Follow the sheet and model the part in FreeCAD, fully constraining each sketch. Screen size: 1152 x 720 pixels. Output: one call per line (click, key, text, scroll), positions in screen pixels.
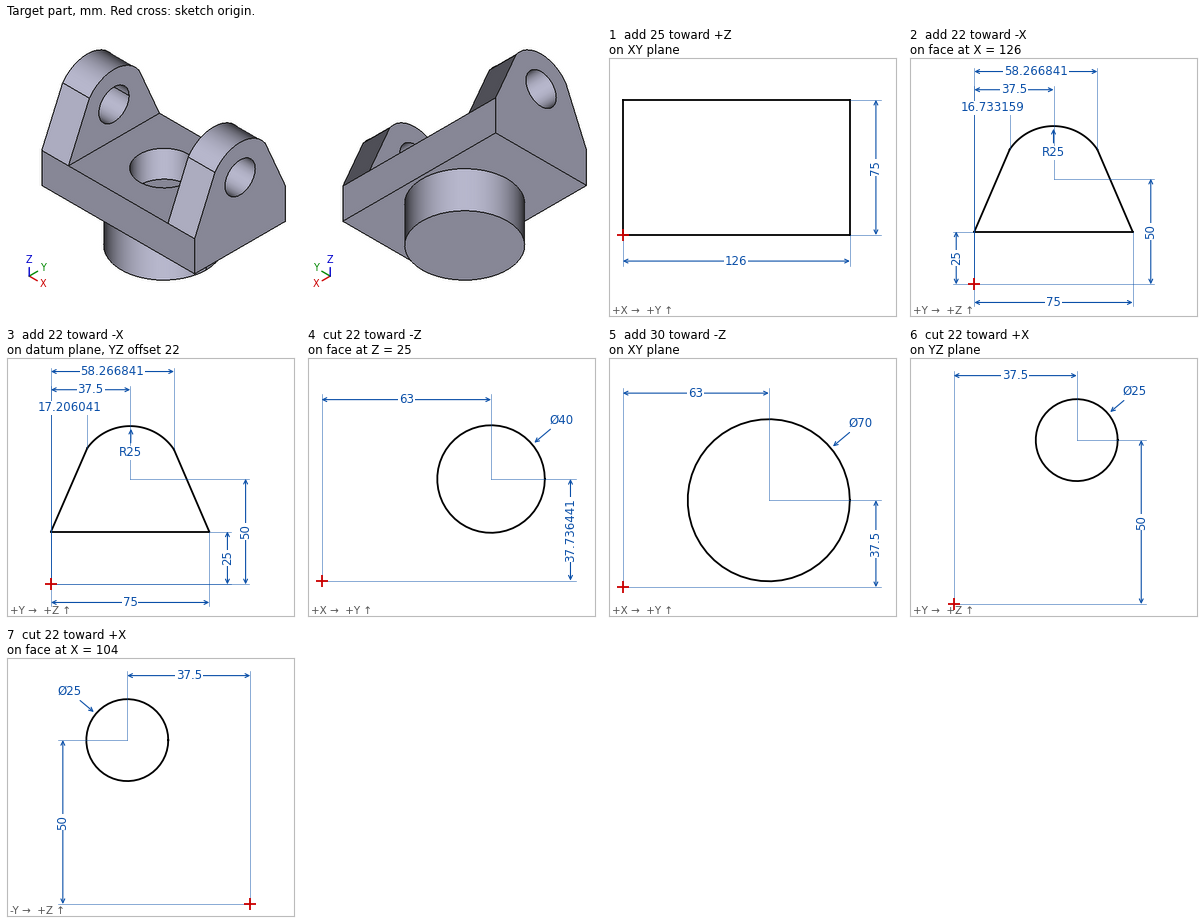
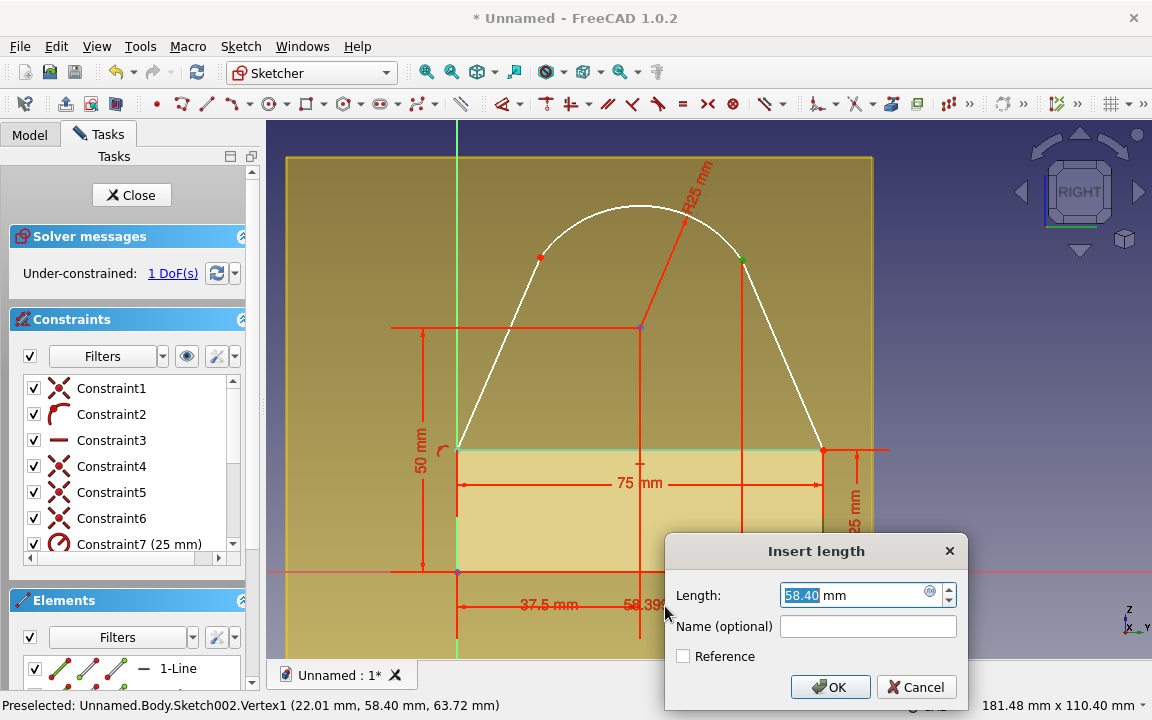
text(58.266841)
key(Return)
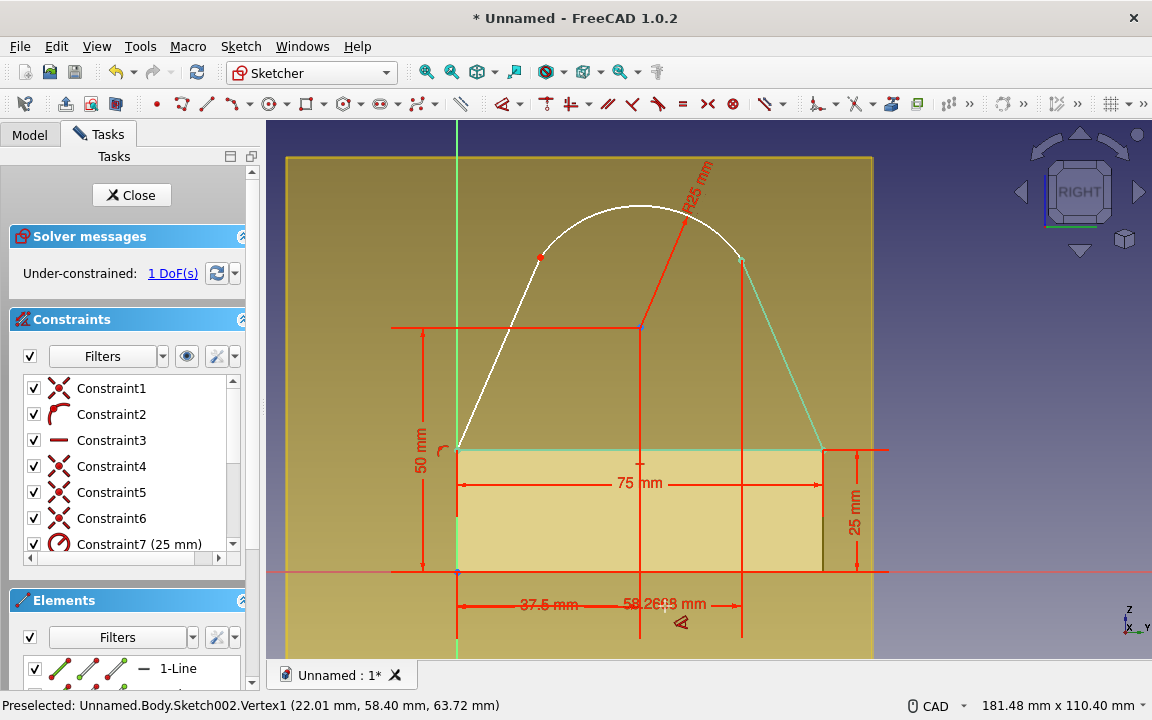
click(540, 258)
click(499, 224)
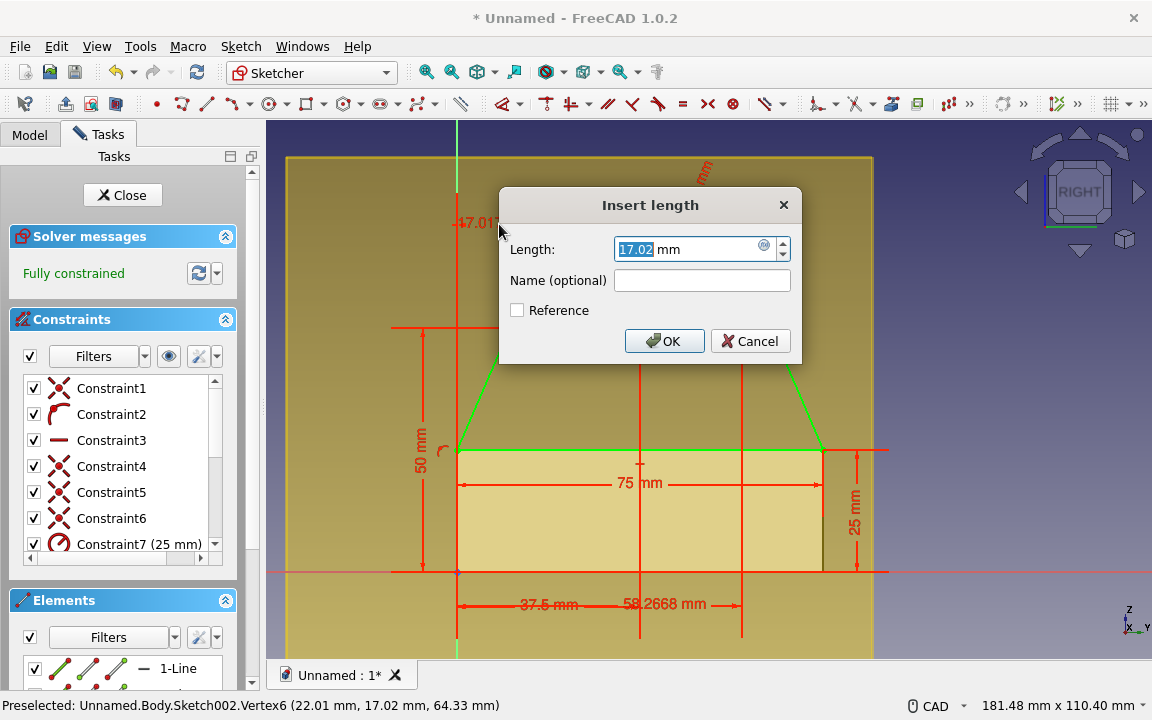
text(17.206041)
key(Return)
key(Escape)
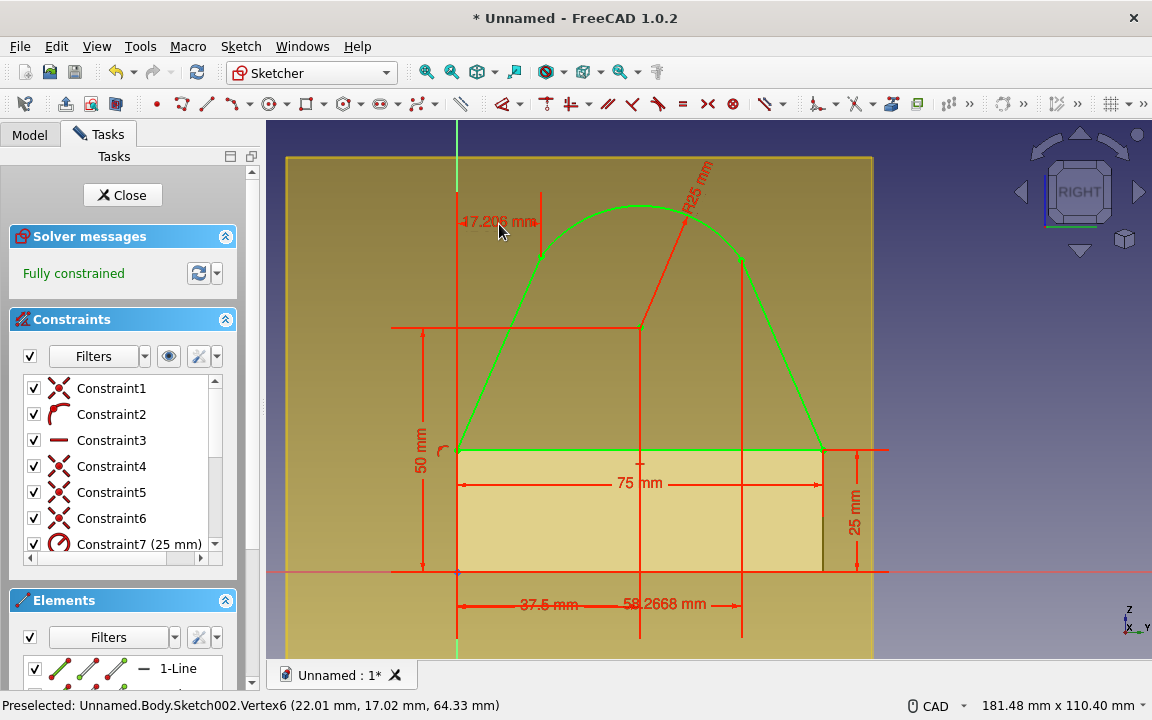
click(123, 195)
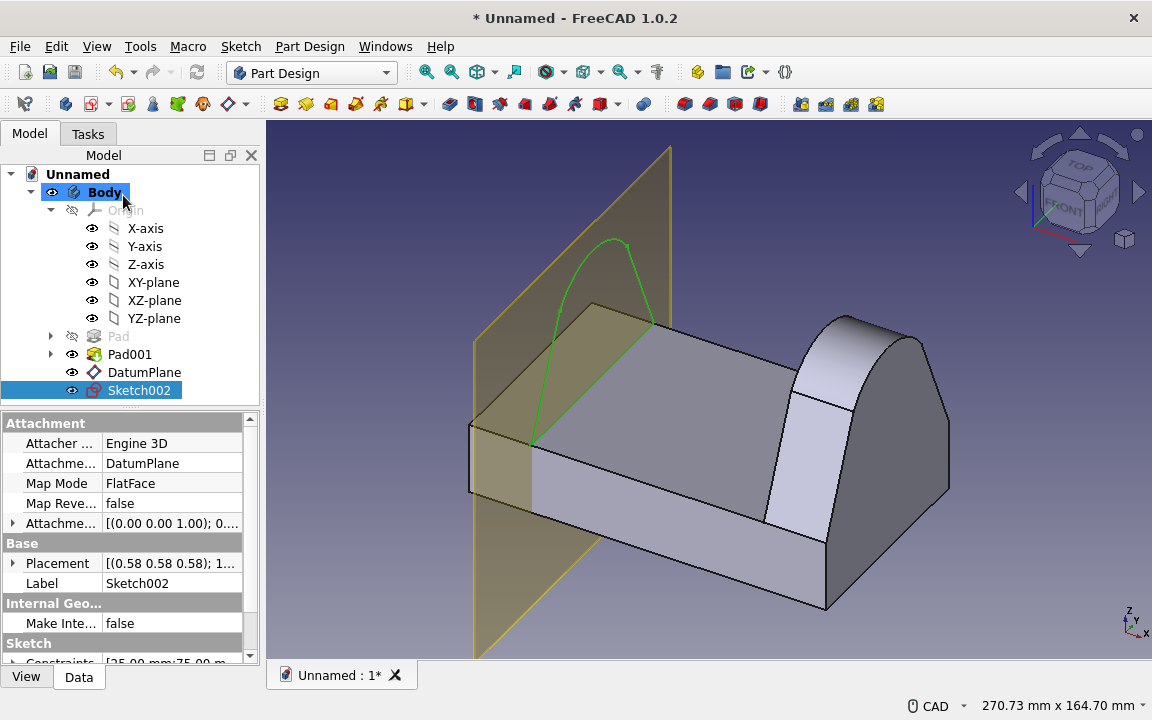
click(281, 104)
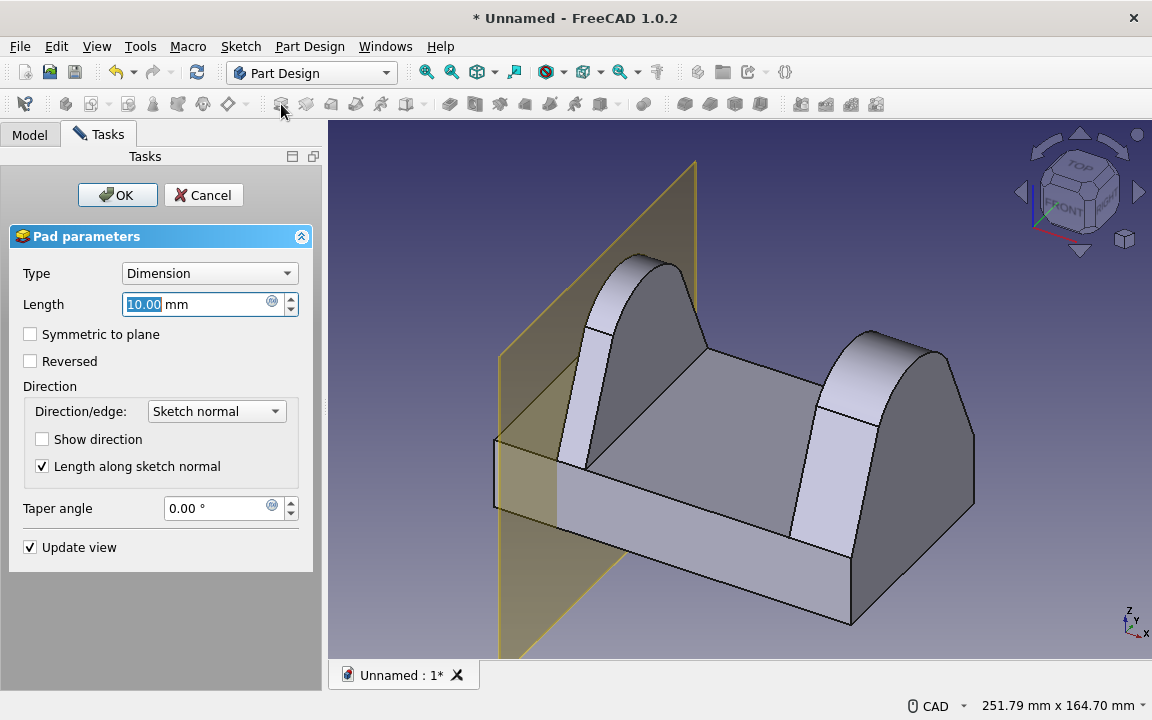
text(22)
key(Tab)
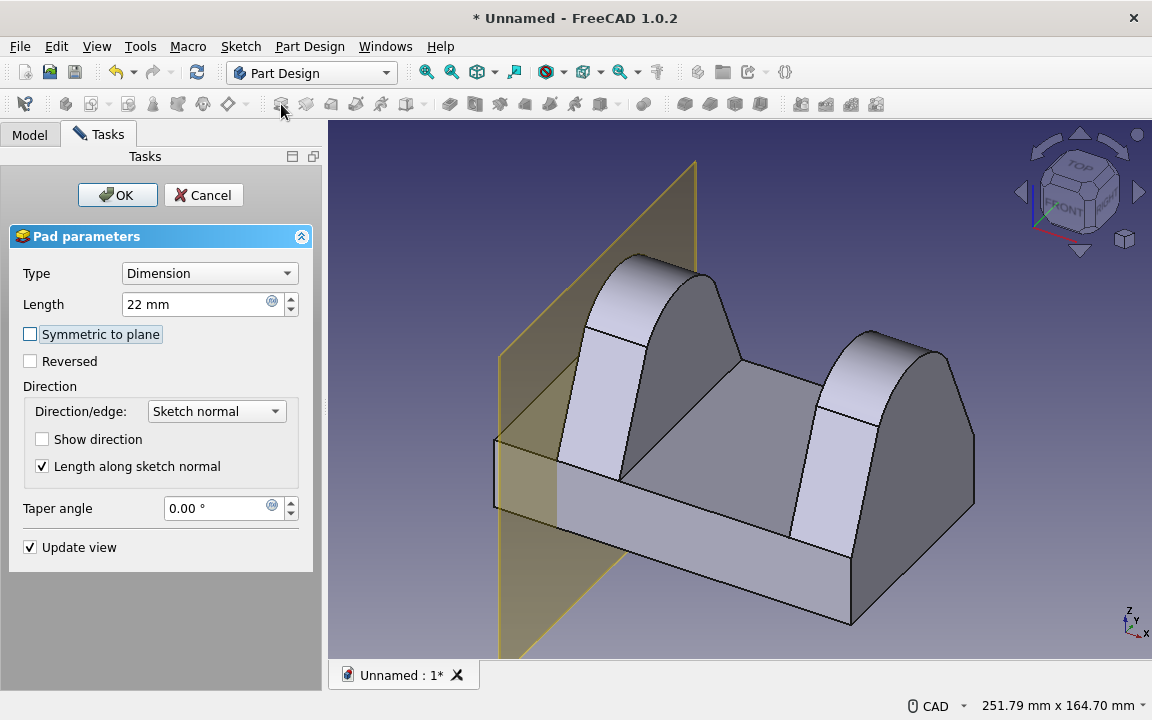
click(31, 361)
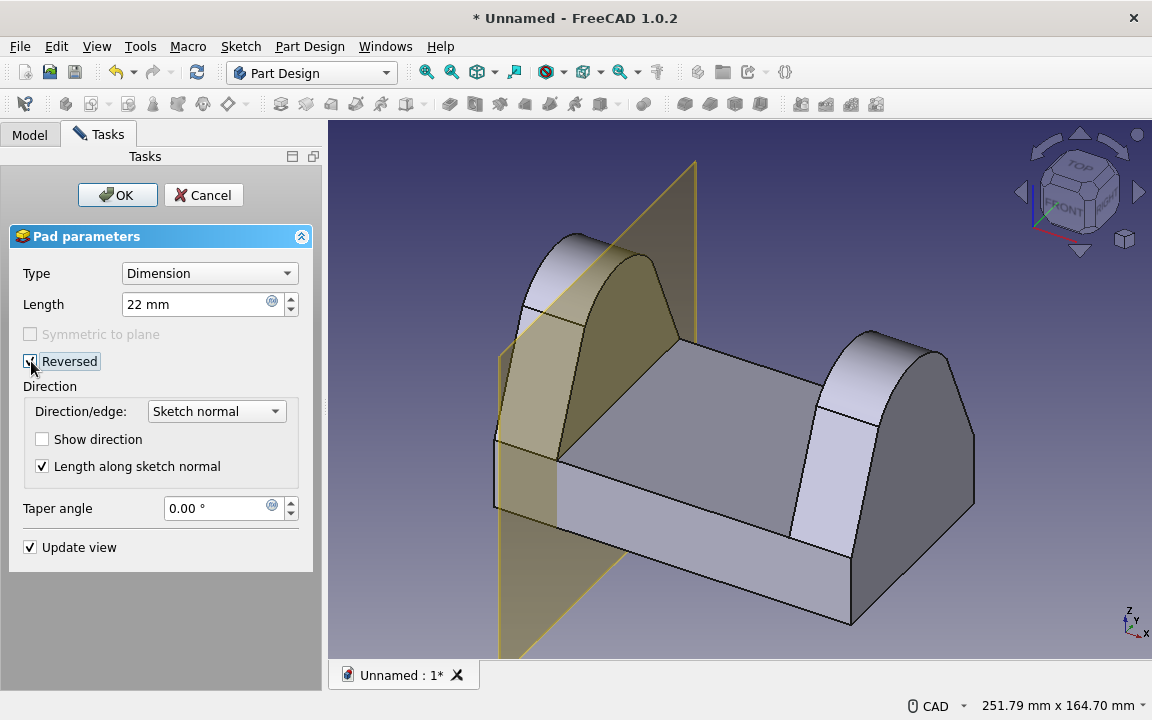
click(118, 195)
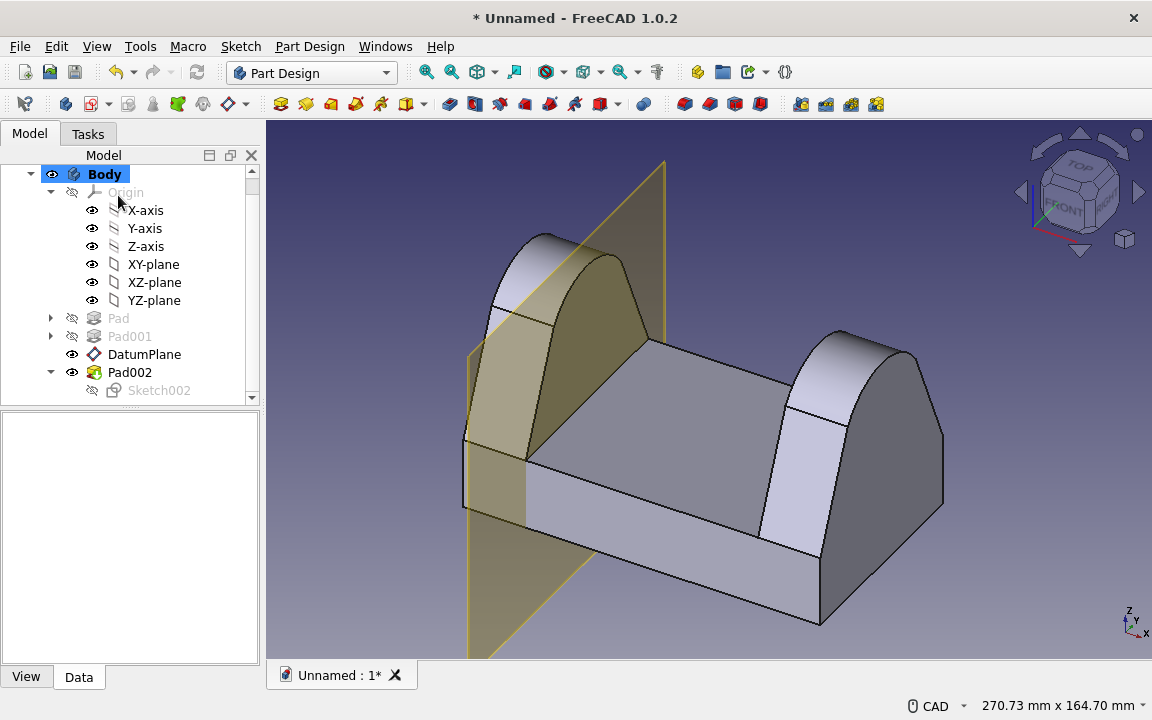
click(117, 354)
key(space)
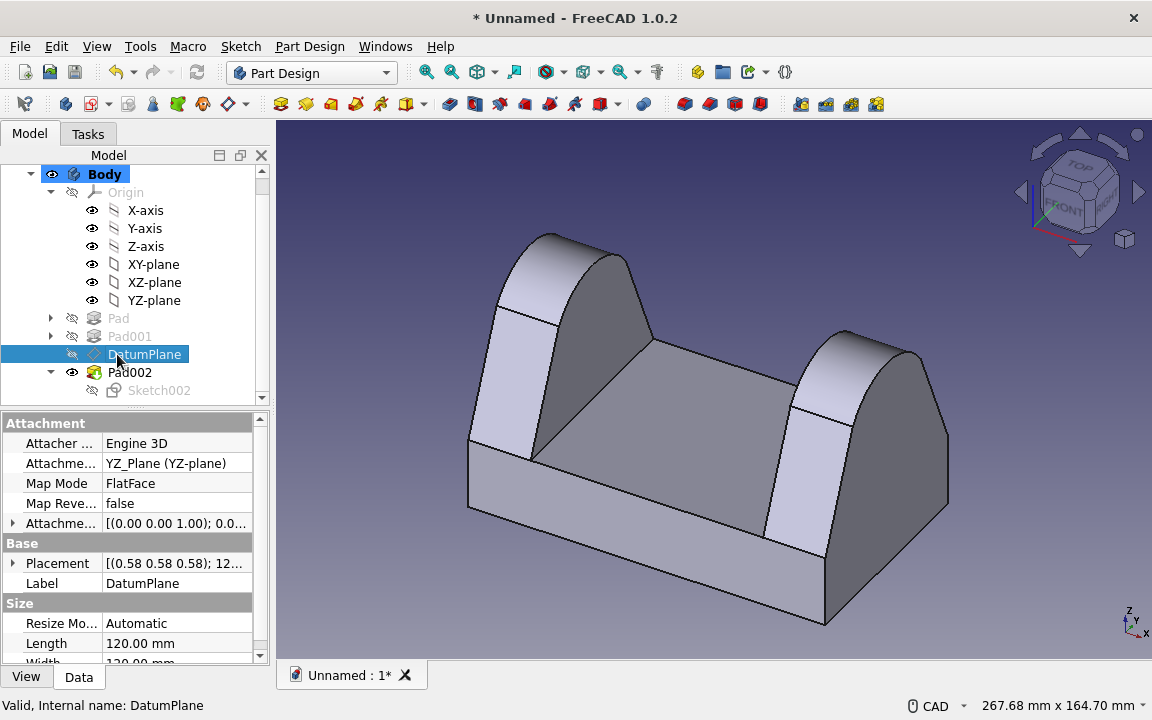
click(708, 437)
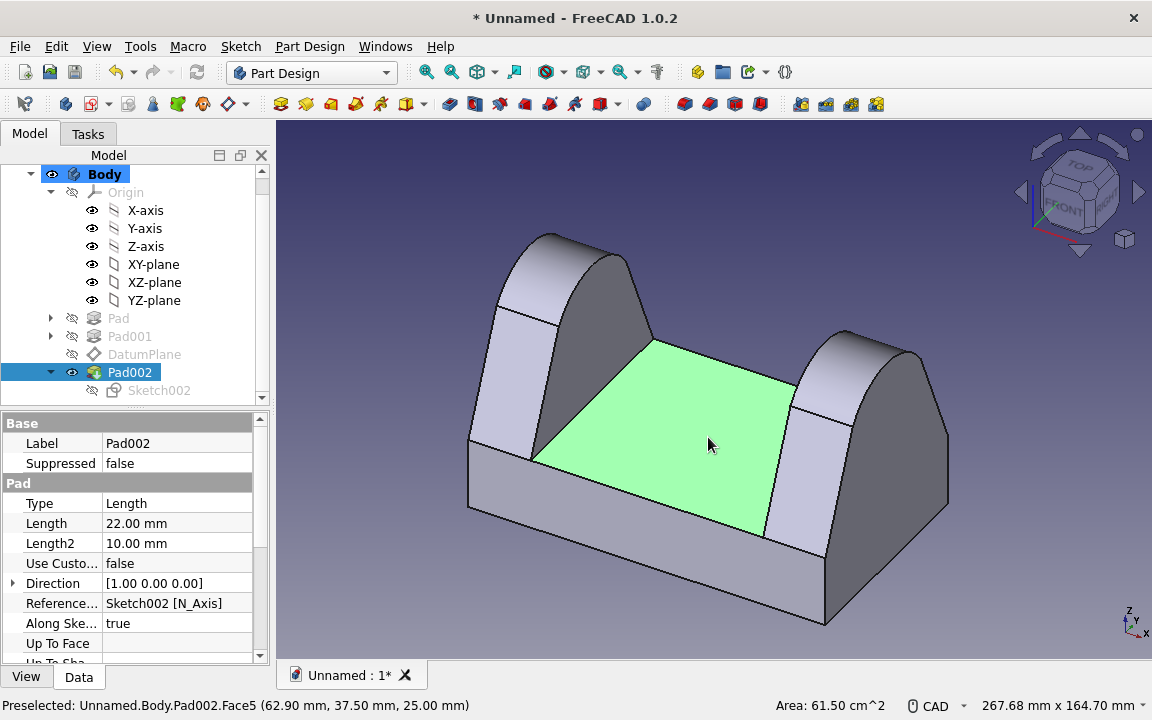
click(90, 104)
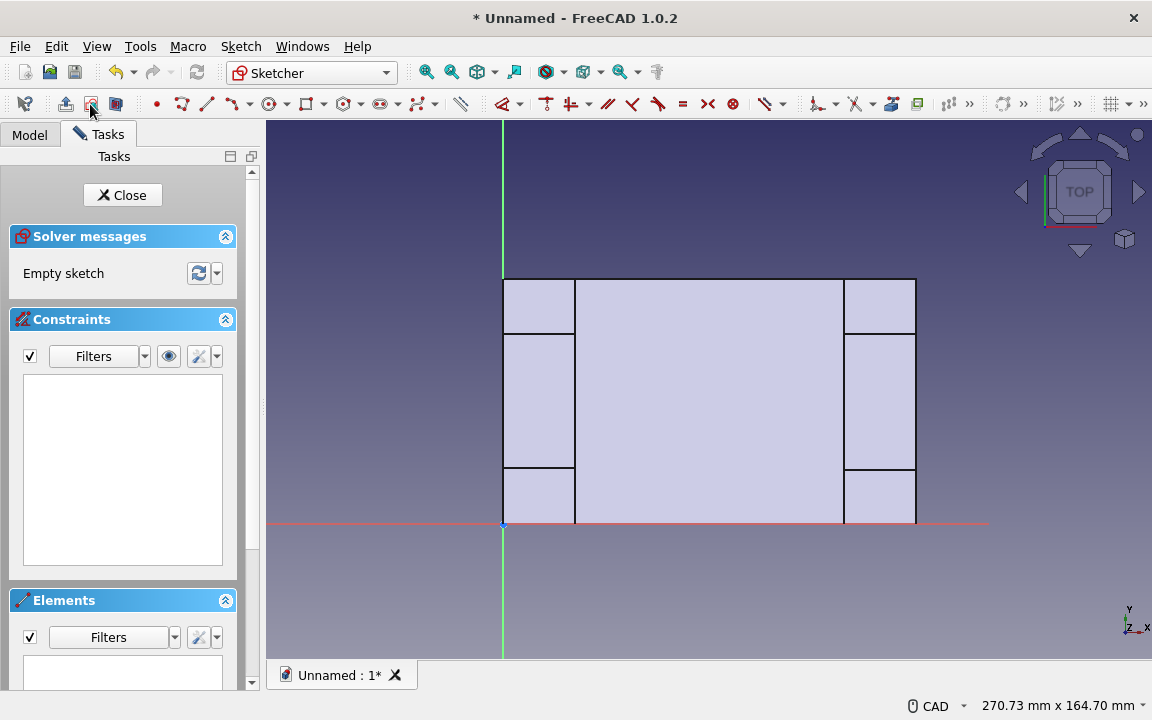
scroll(637, 479, up, 3)